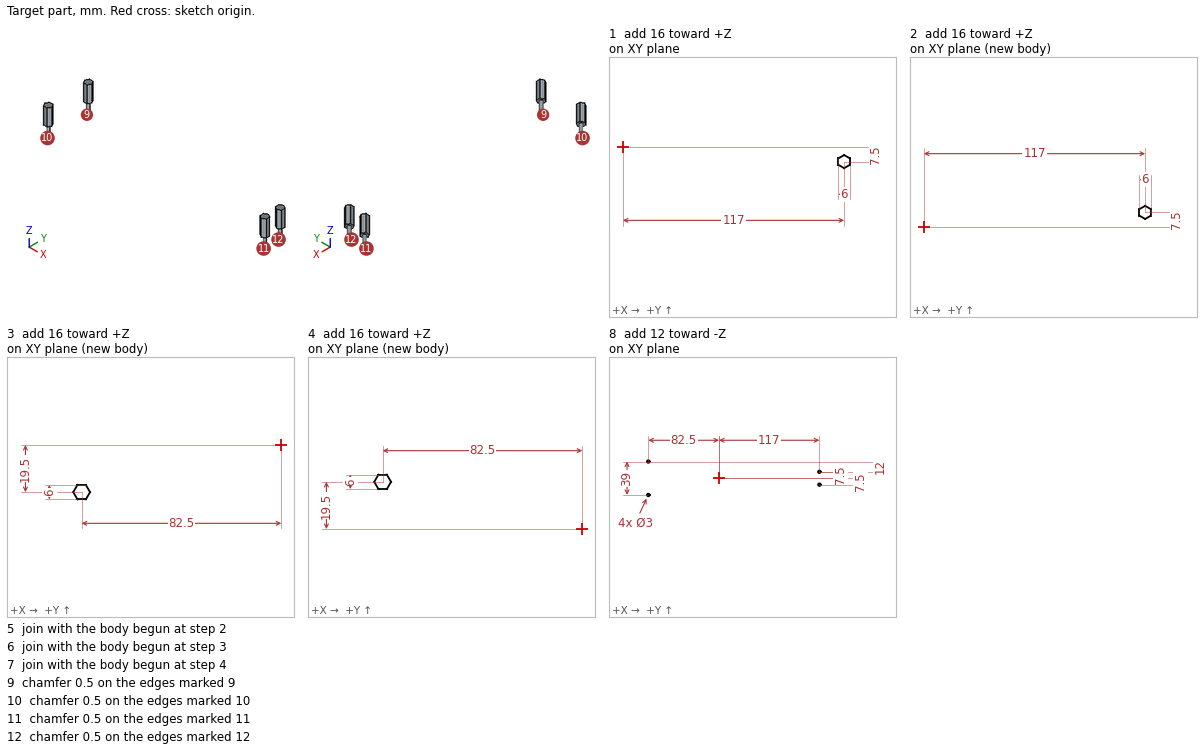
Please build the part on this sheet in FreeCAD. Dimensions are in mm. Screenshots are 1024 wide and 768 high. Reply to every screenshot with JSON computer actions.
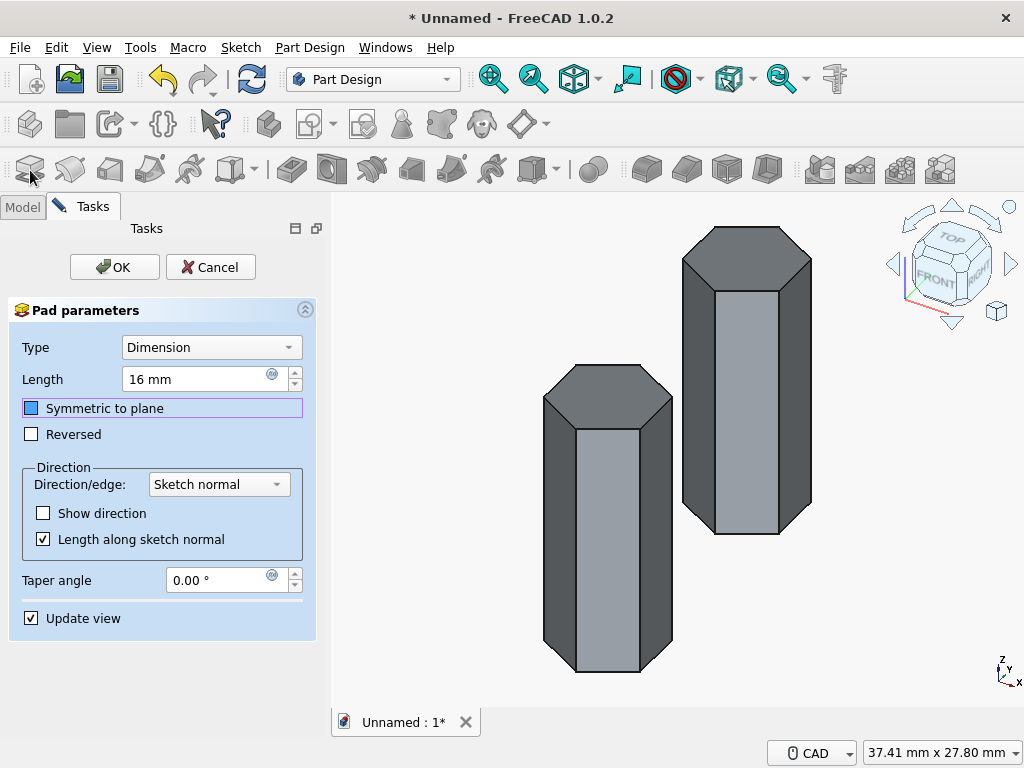
{"action": "left_click", "coordinate": [115, 267]}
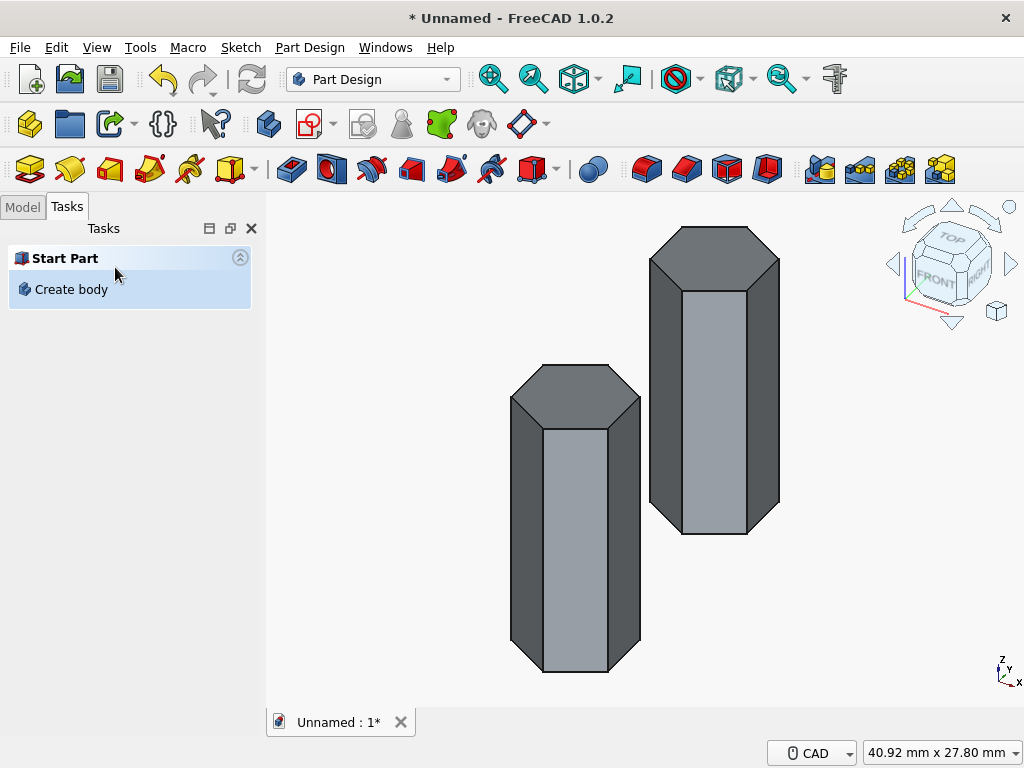
{"action": "left_click", "coordinate": [494, 80]}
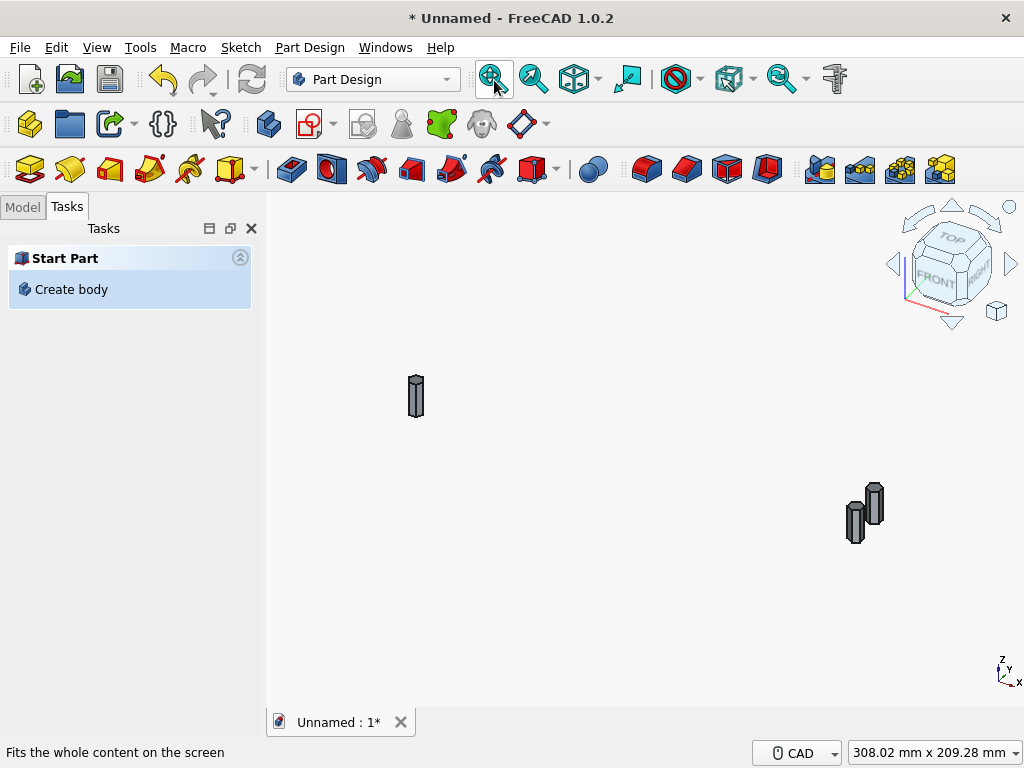
{"action": "left_click", "coordinate": [270, 124]}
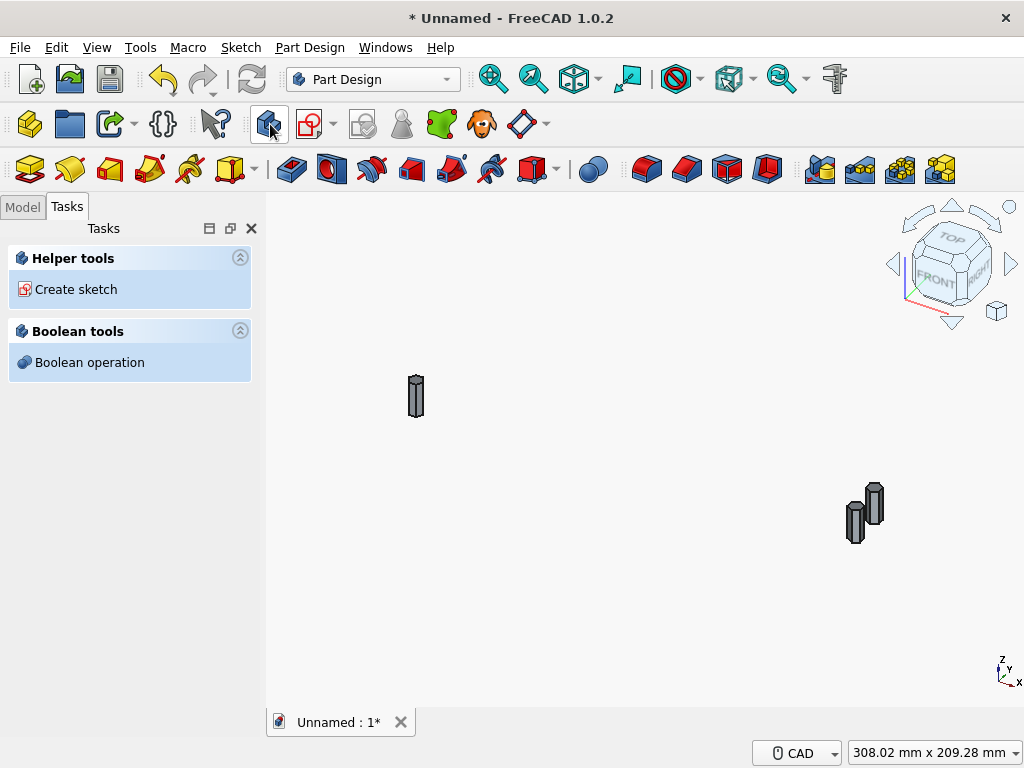
{"action": "left_click", "coordinate": [306, 667]}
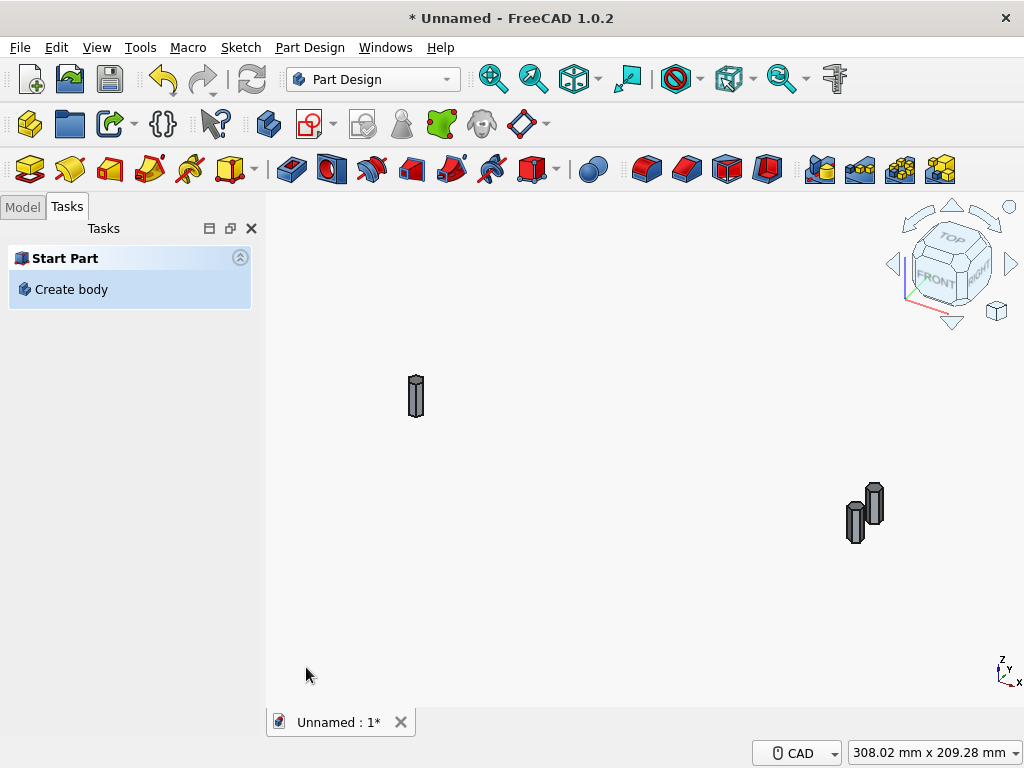
{"action": "left_click", "coordinate": [310, 124]}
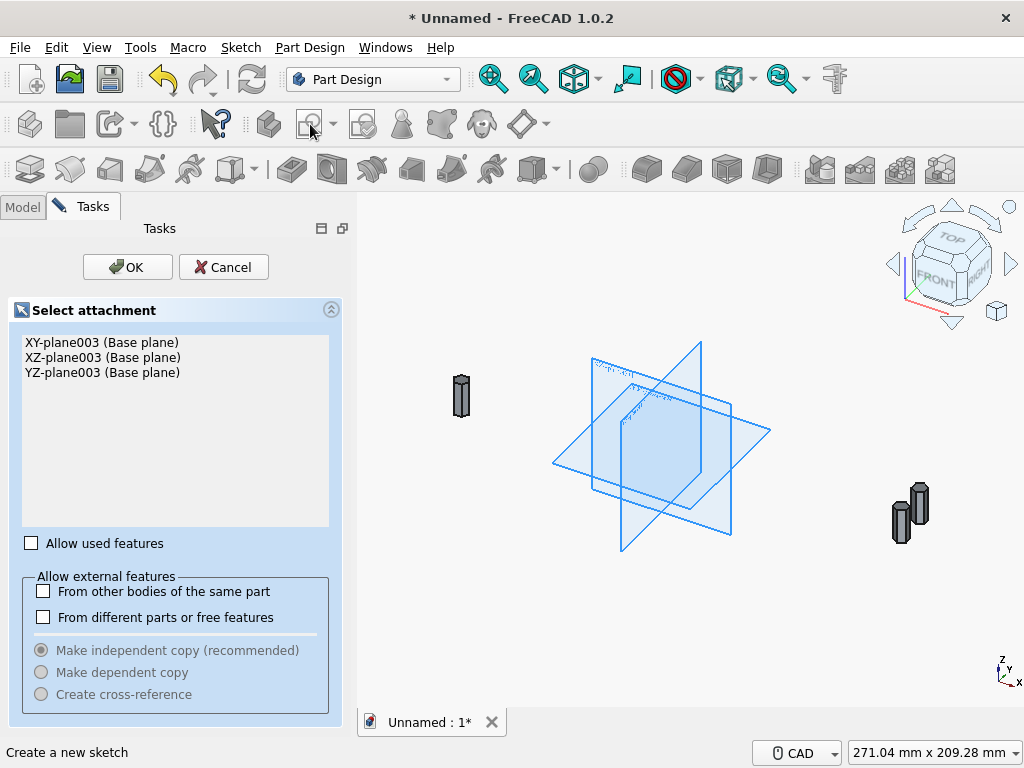
{"action": "left_click", "coordinate": [82, 342]}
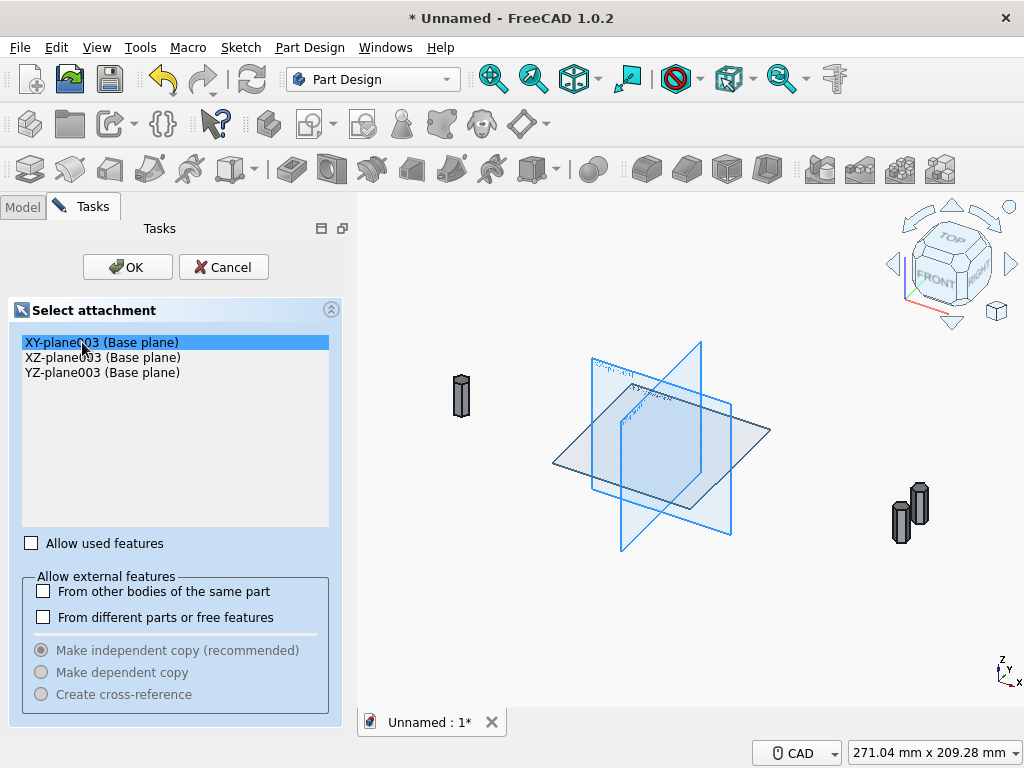
{"action": "left_click", "coordinate": [128, 267]}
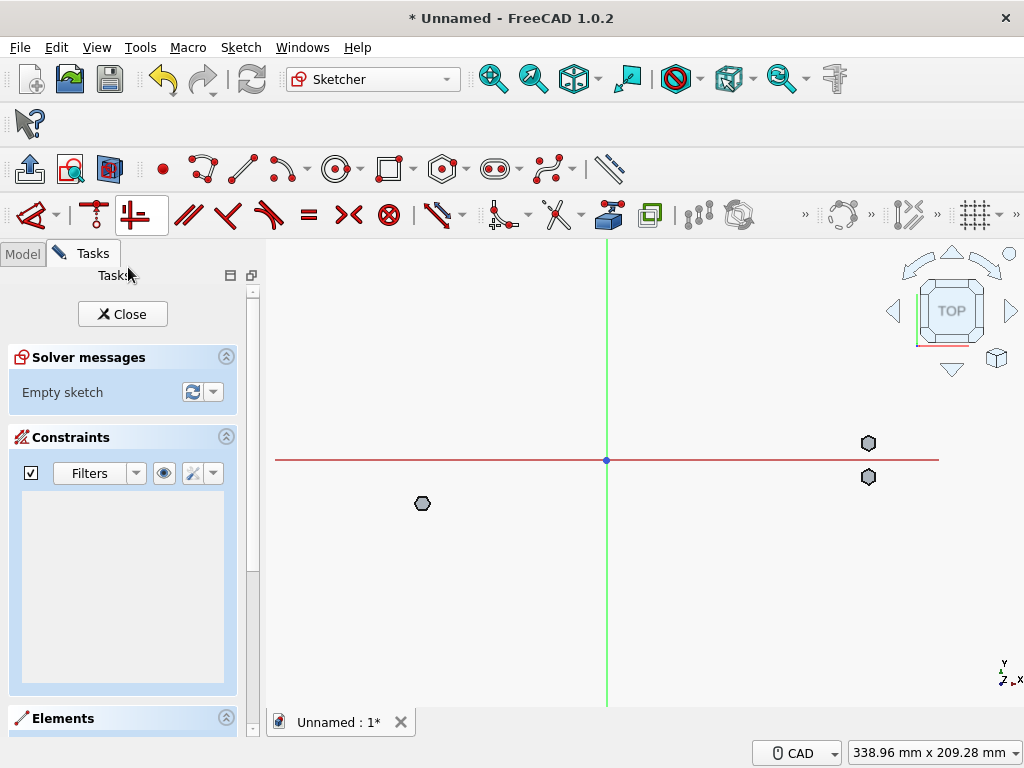
{"action": "scroll", "coordinate": [414, 414], "scroll_direction": "up", "scroll_amount": 15}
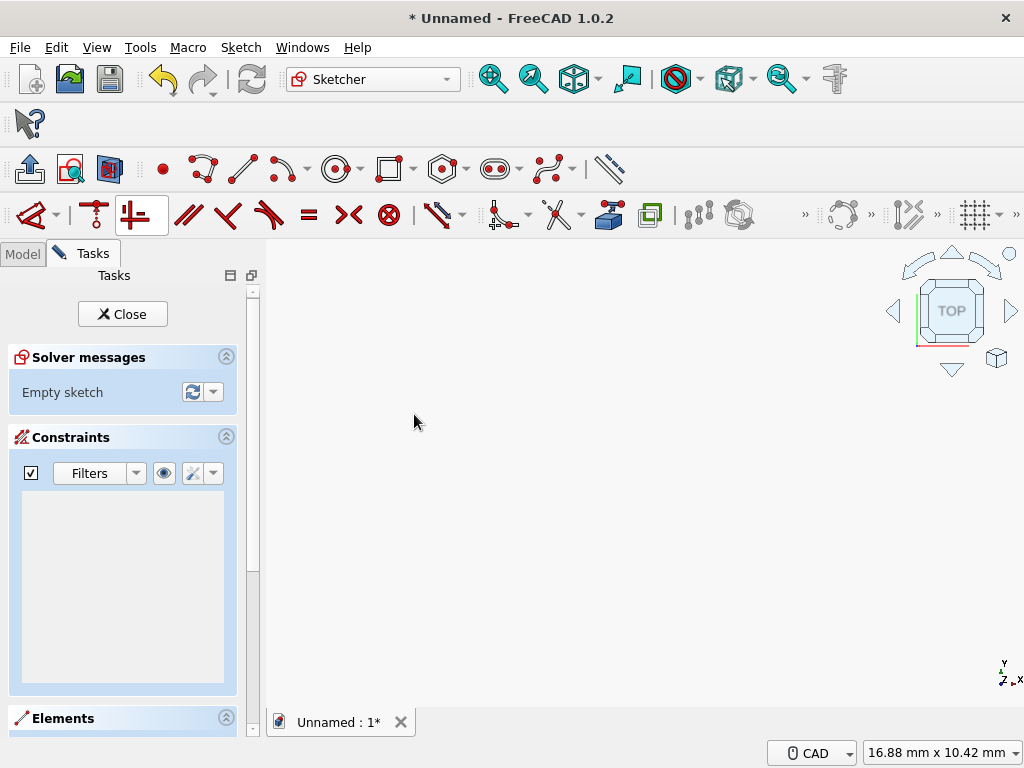
{"action": "left_click", "coordinate": [442, 170]}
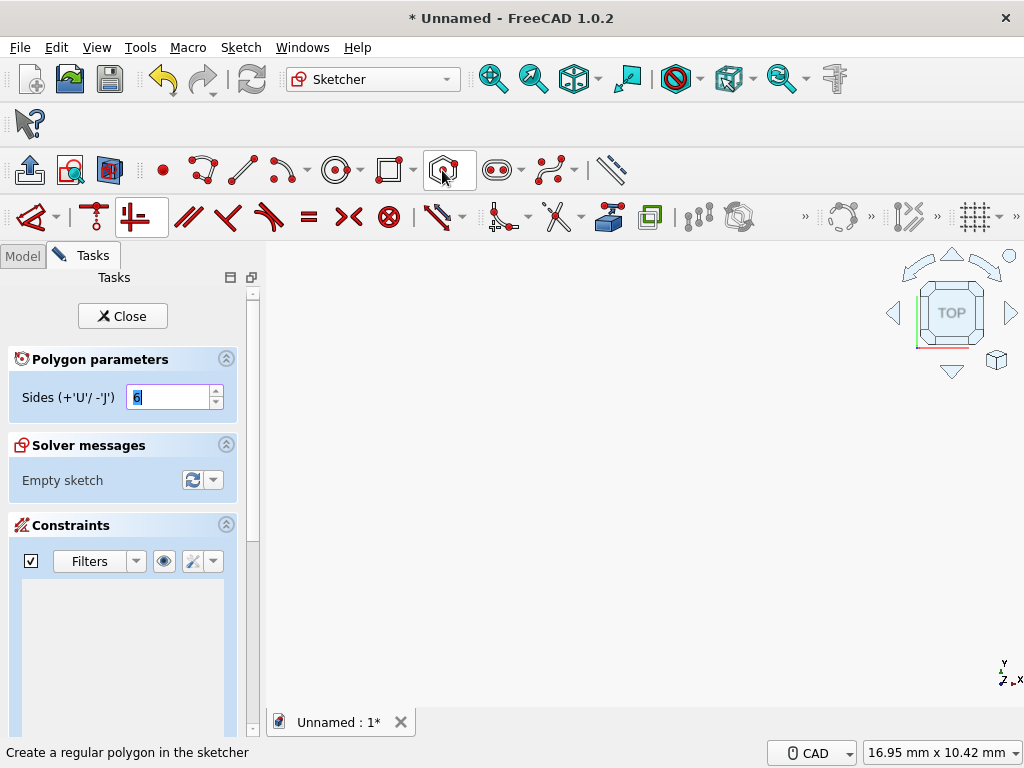
{"action": "left_click", "coordinate": [580, 458]}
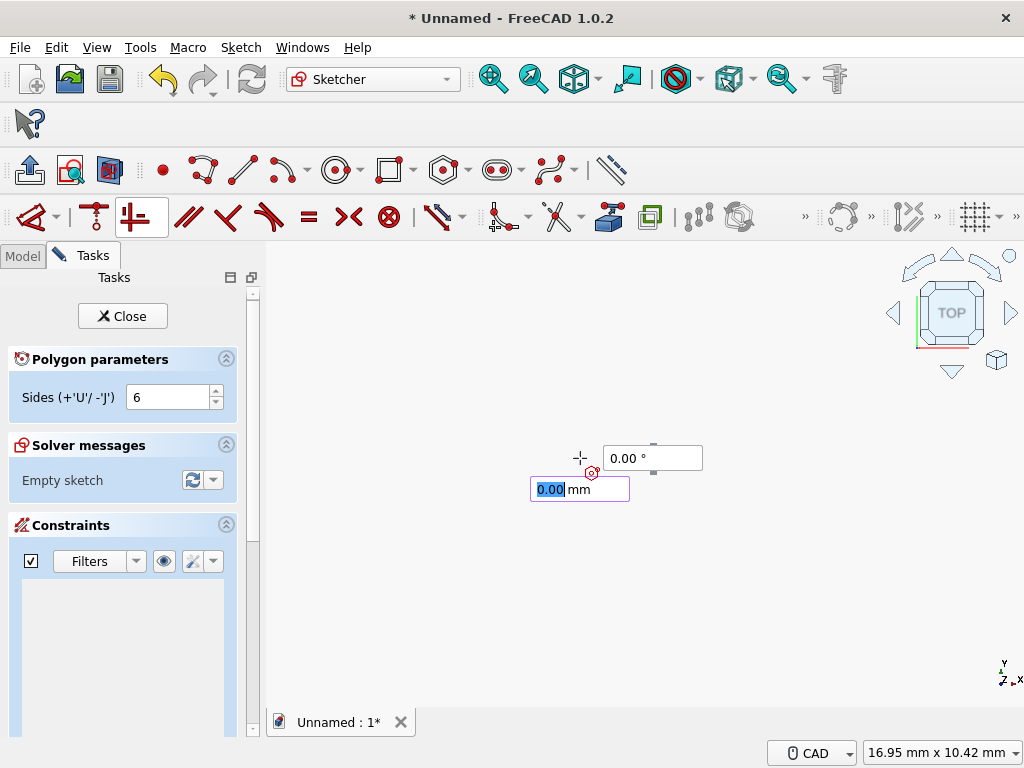
{"action": "left_click", "coordinate": [735, 458]}
{"action": "right_click", "coordinate": [735, 458]}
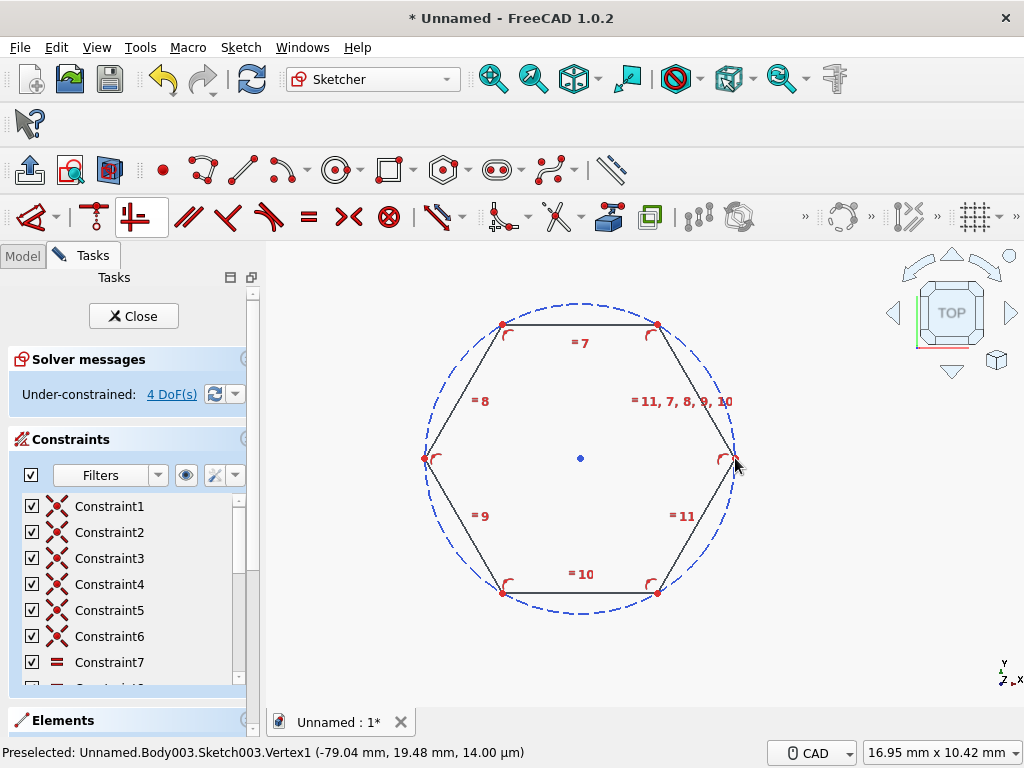
{"action": "left_click", "coordinate": [611, 325]}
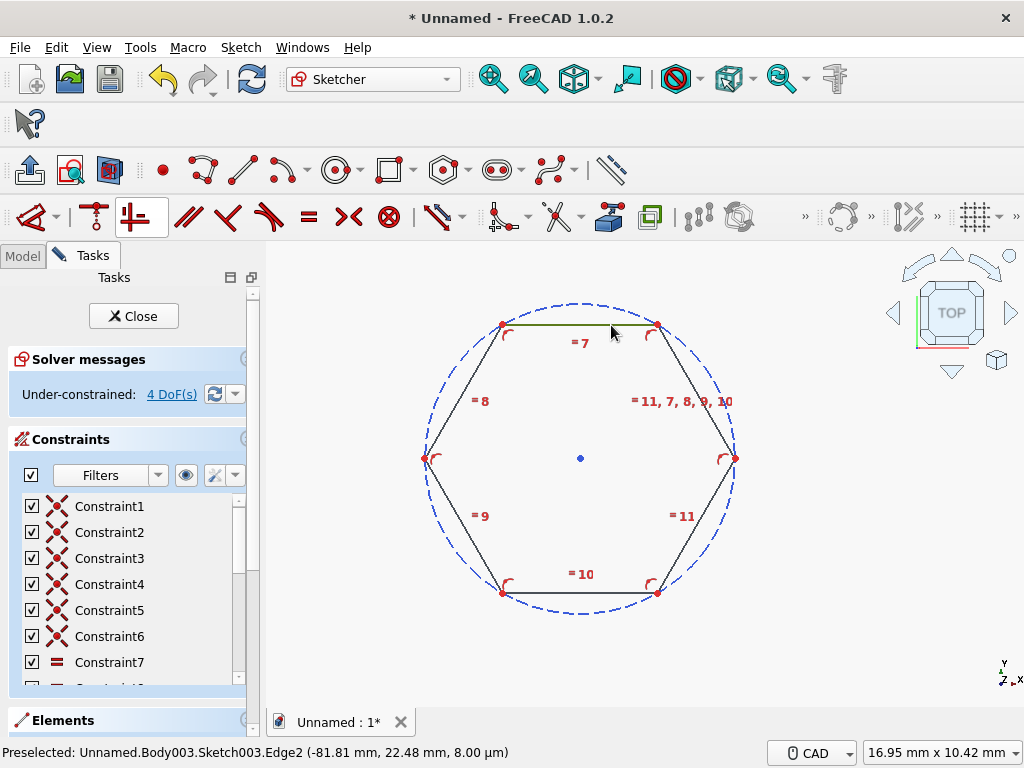
{"action": "key", "text": "h"}